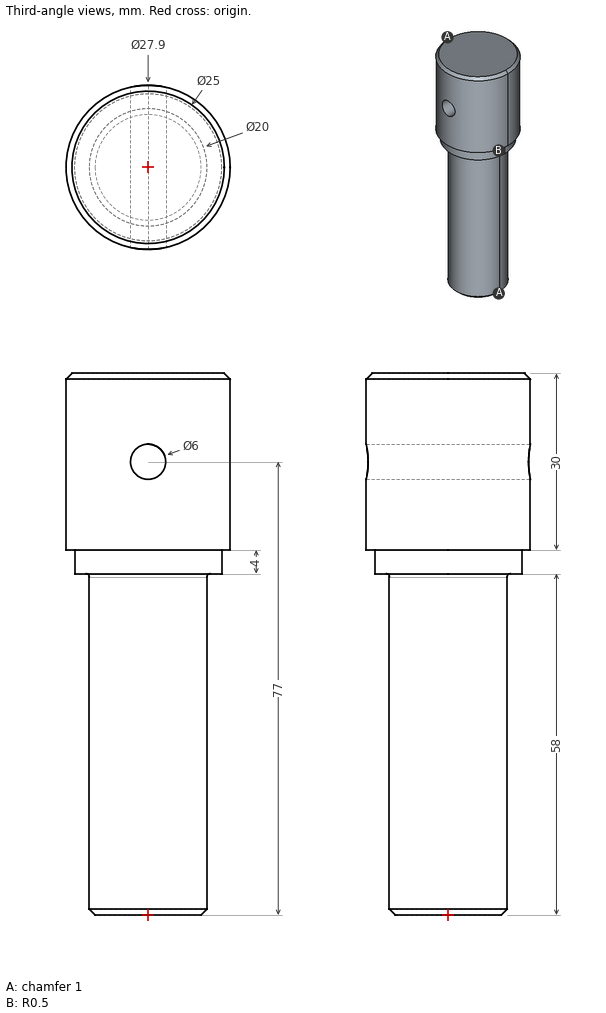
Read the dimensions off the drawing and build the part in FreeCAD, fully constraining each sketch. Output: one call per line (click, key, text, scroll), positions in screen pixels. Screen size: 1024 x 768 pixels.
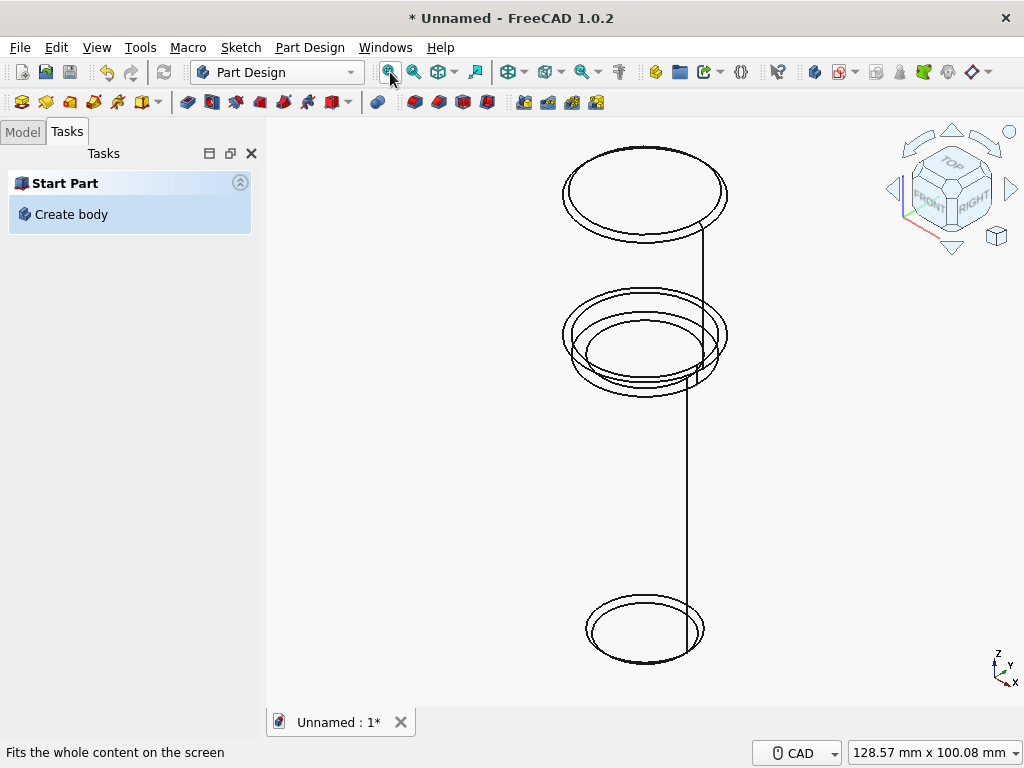
click(603, 329)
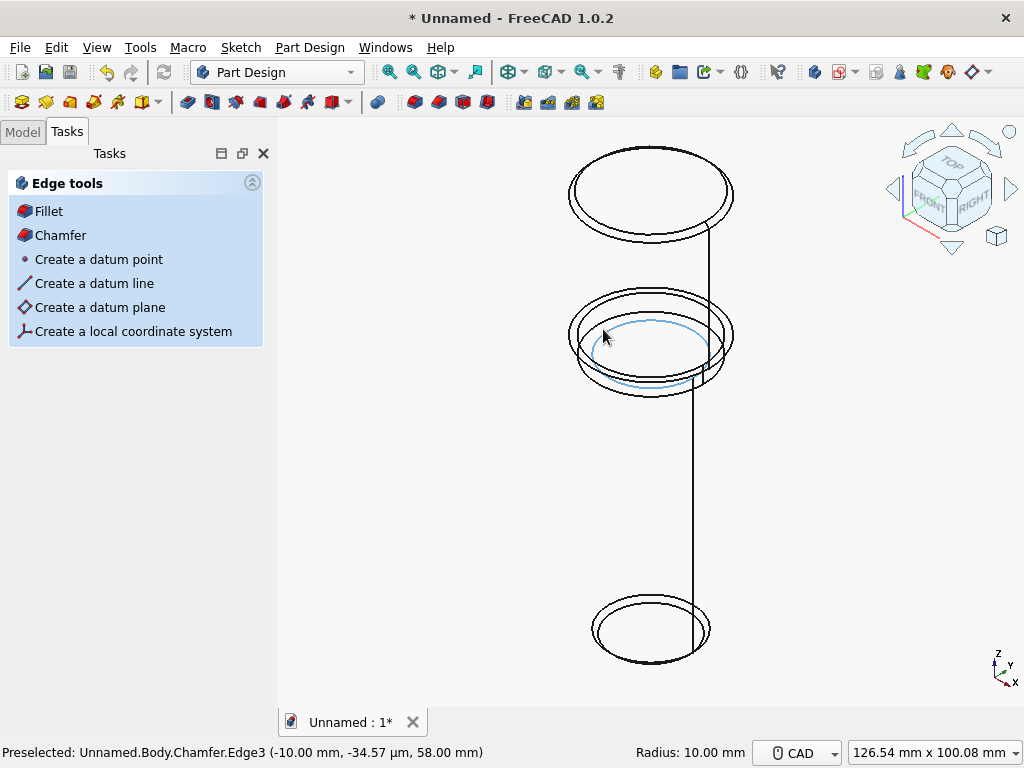
key(v)
key(1)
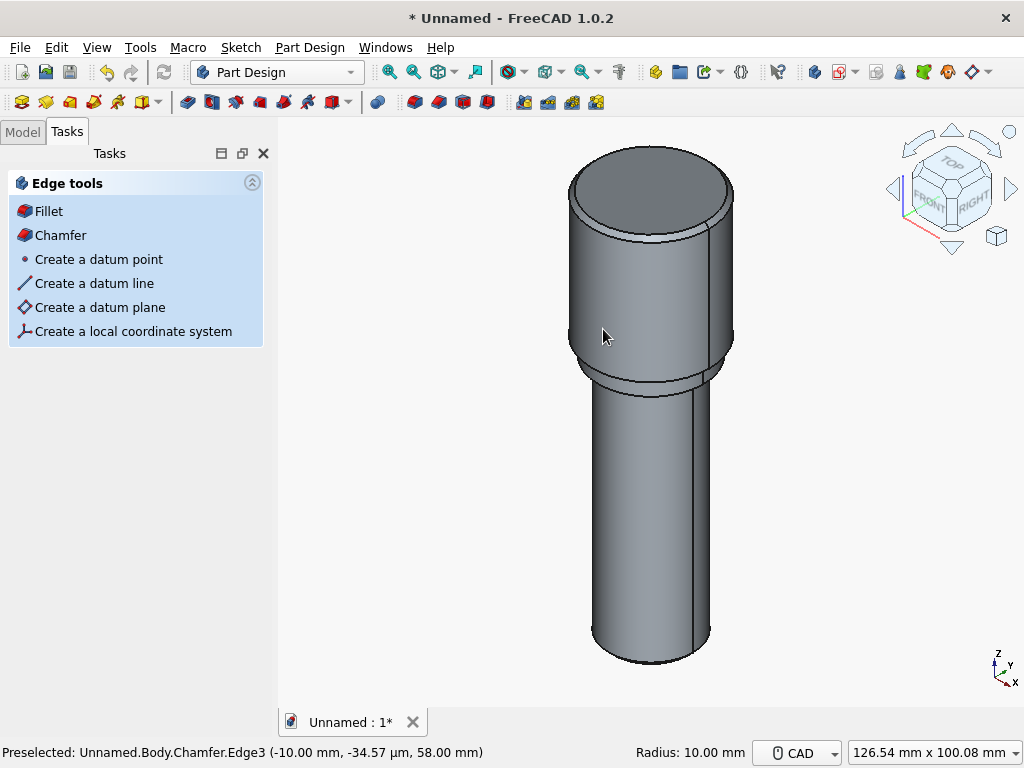
click(416, 102)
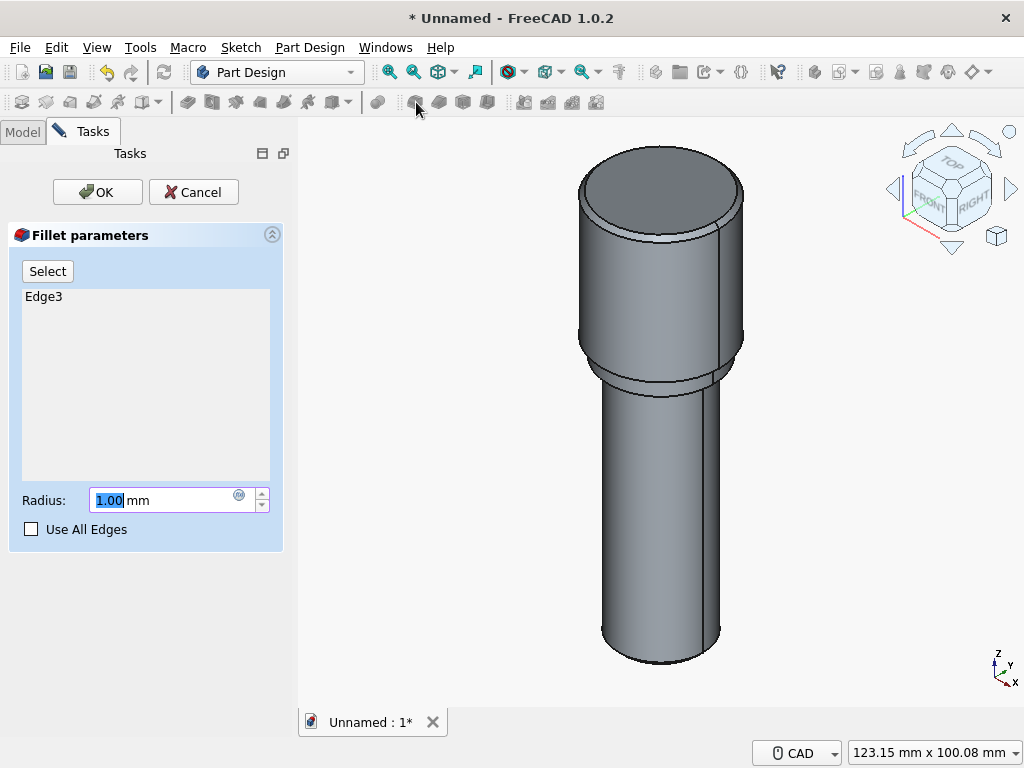
text(0.5)
key(Tab)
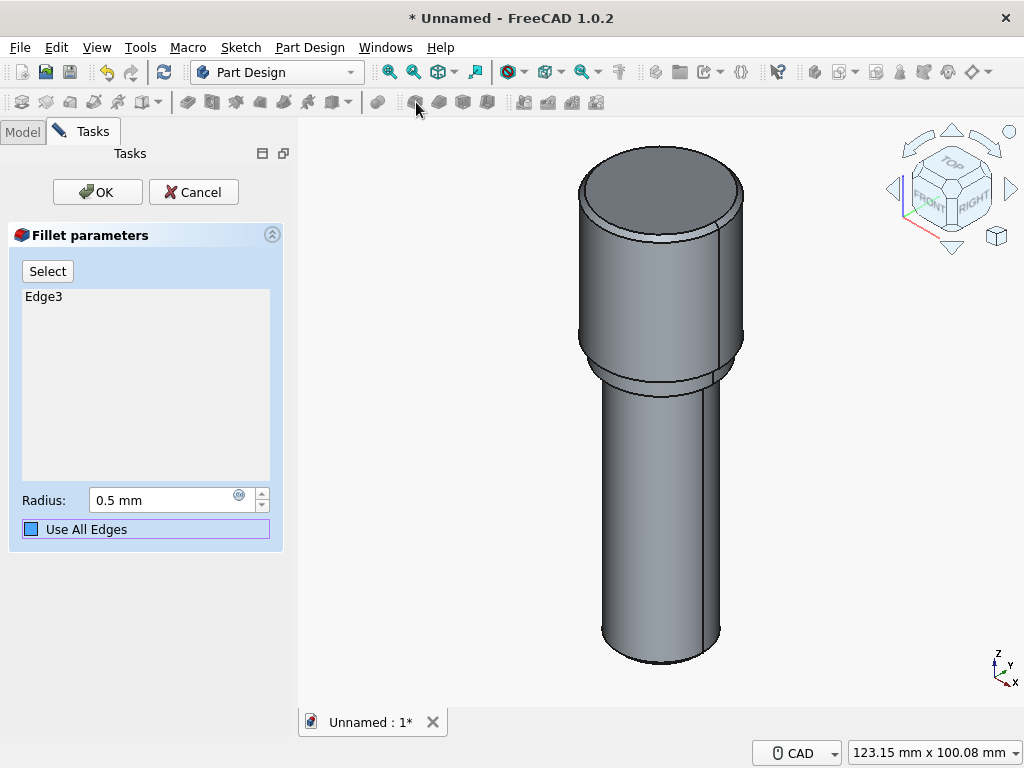
click(98, 192)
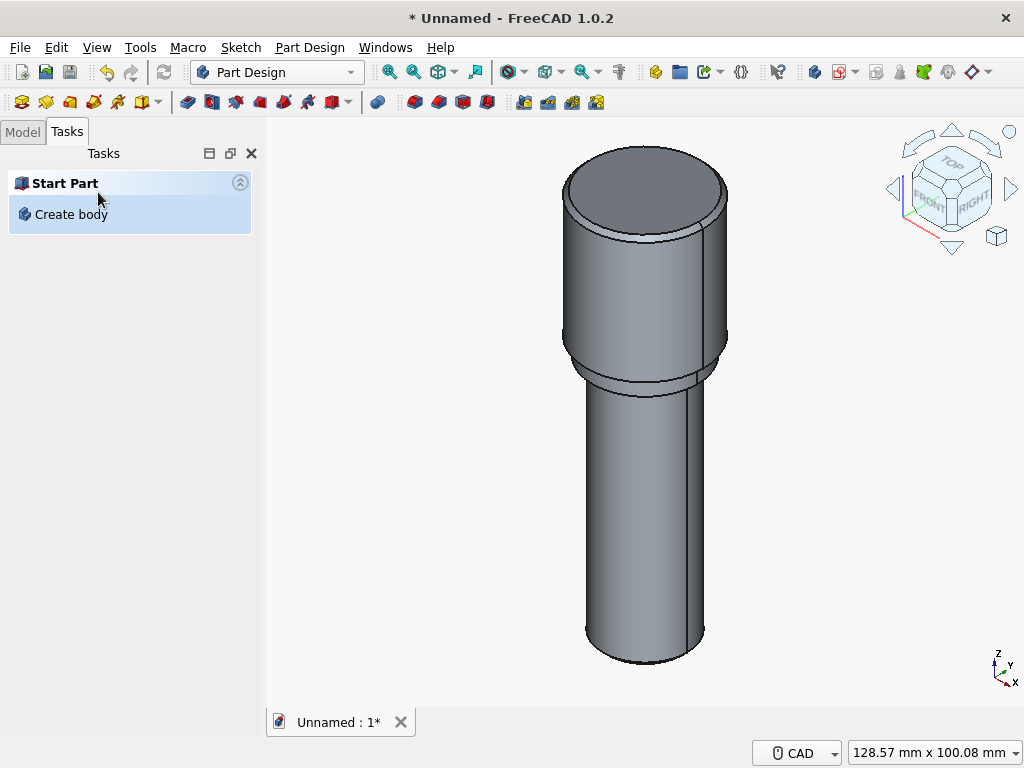
click(840, 72)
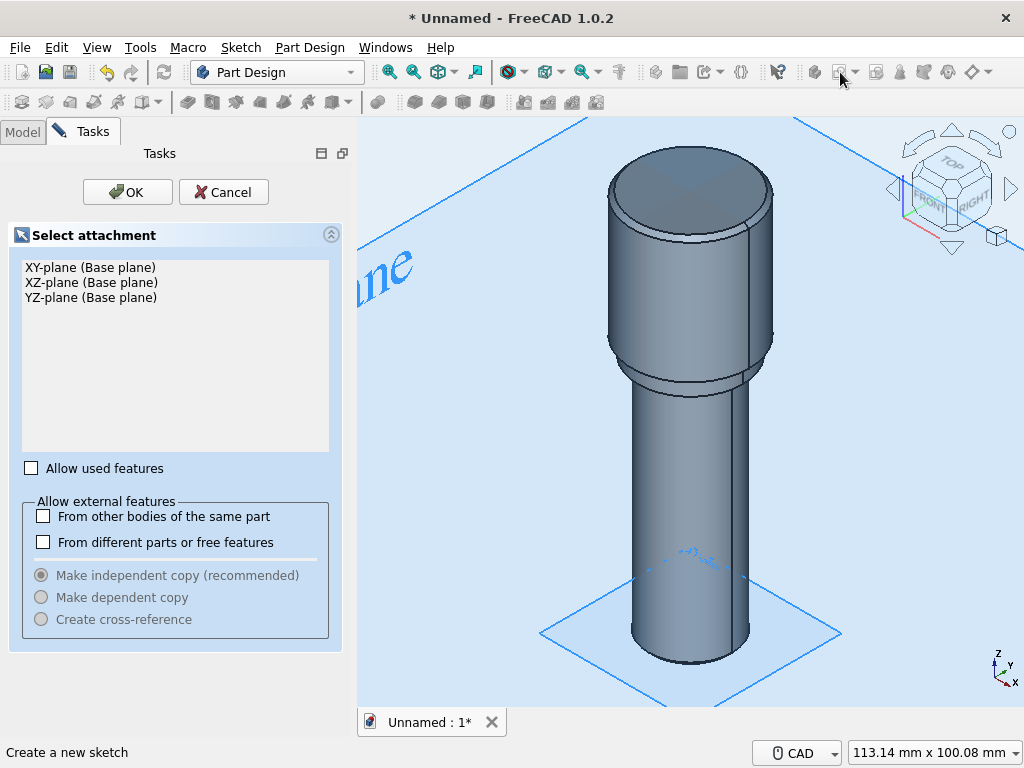
click(82, 282)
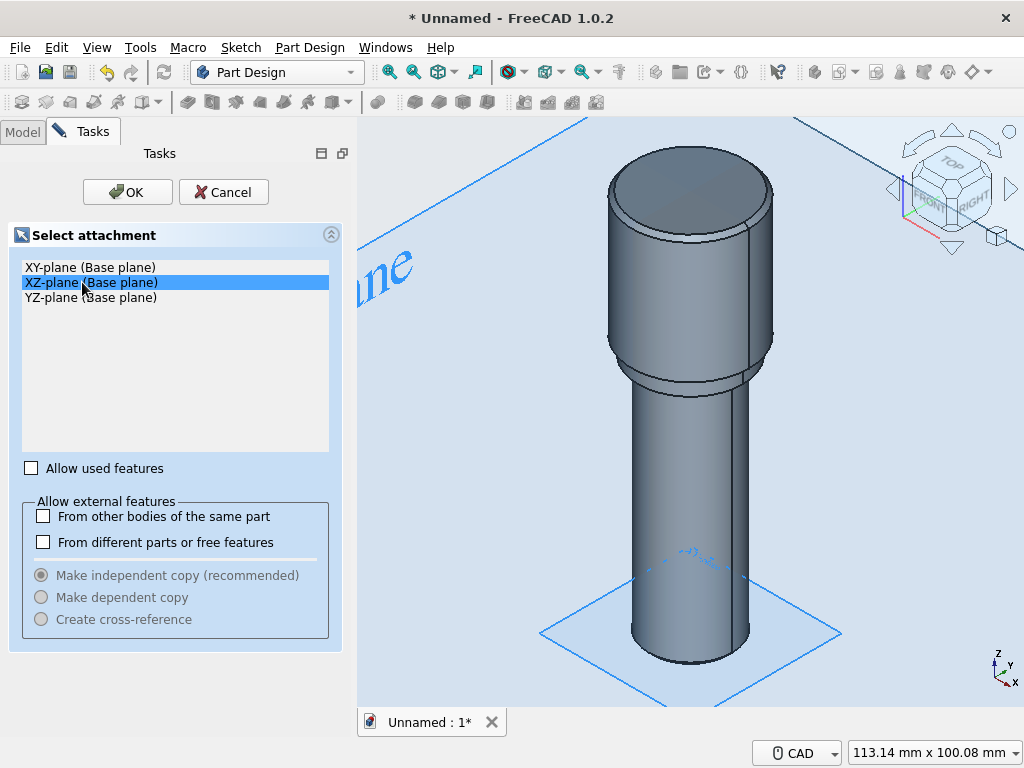
click(128, 192)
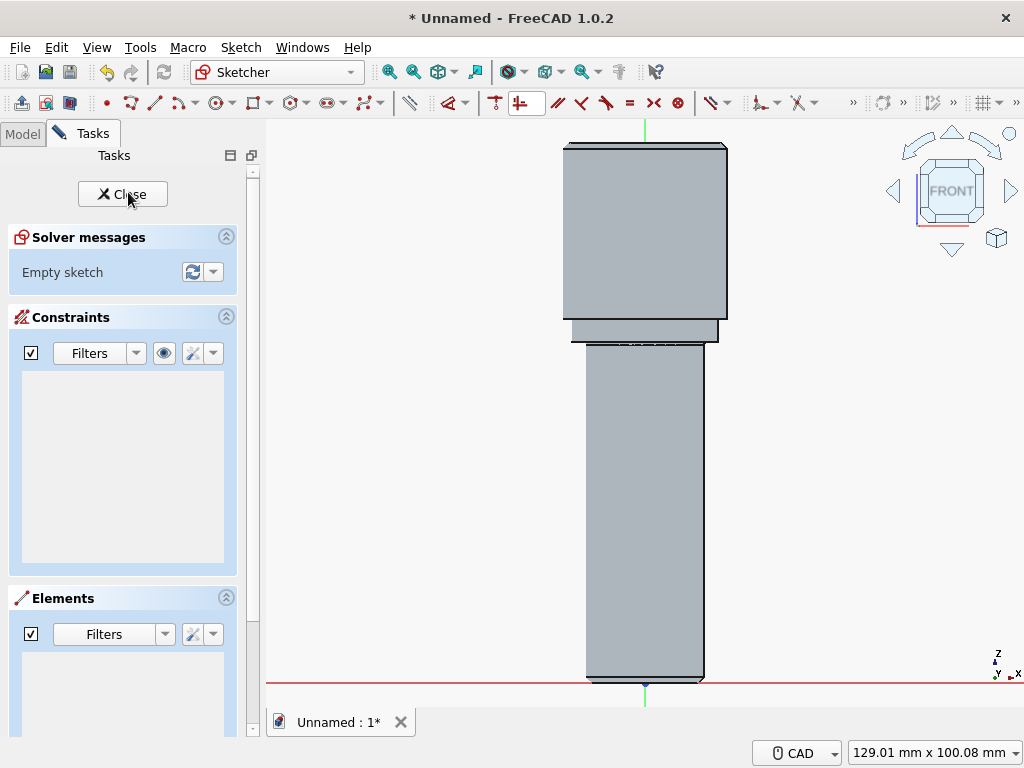
click(70, 104)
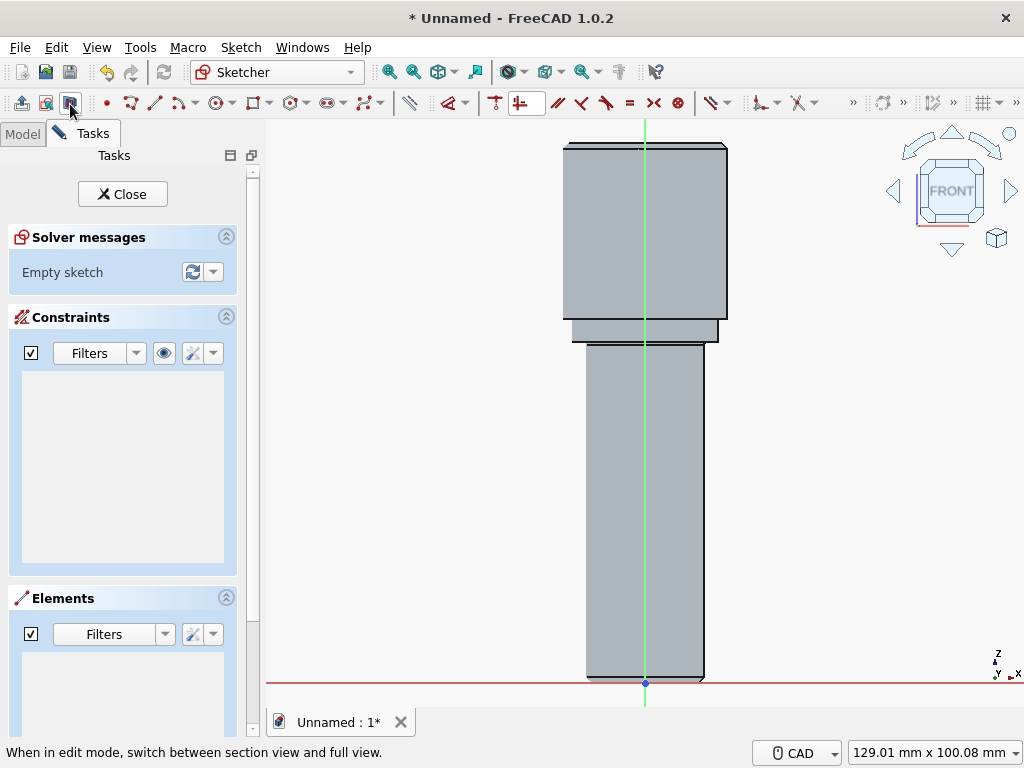
scroll(652, 213, up, 12)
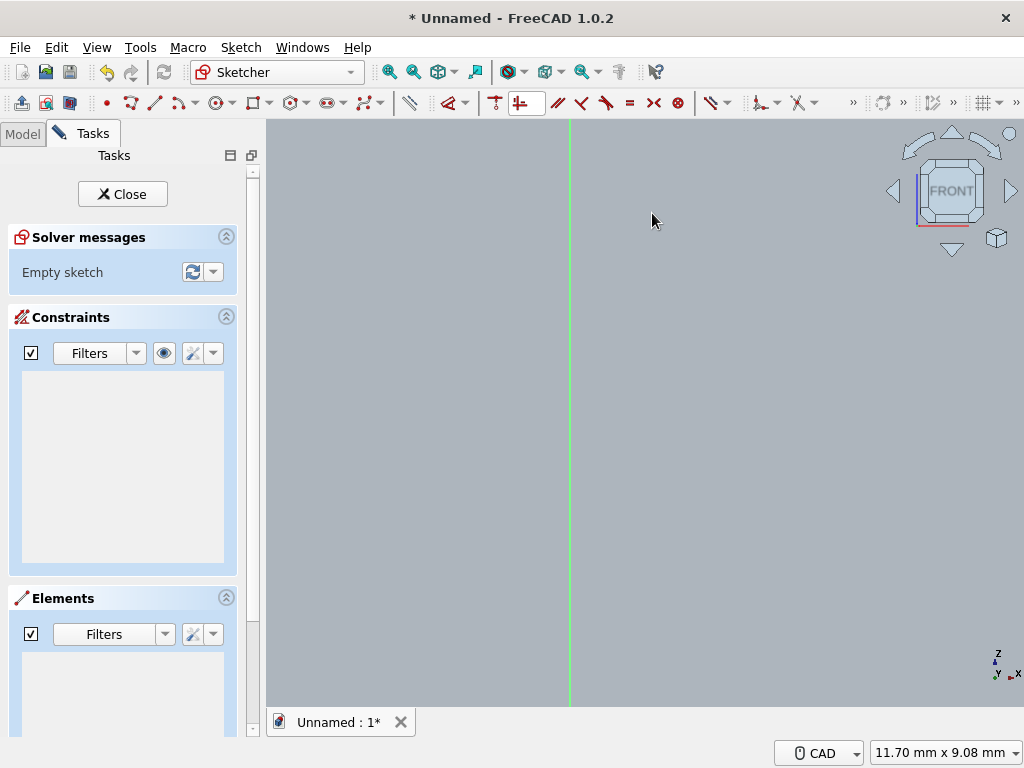
click(216, 104)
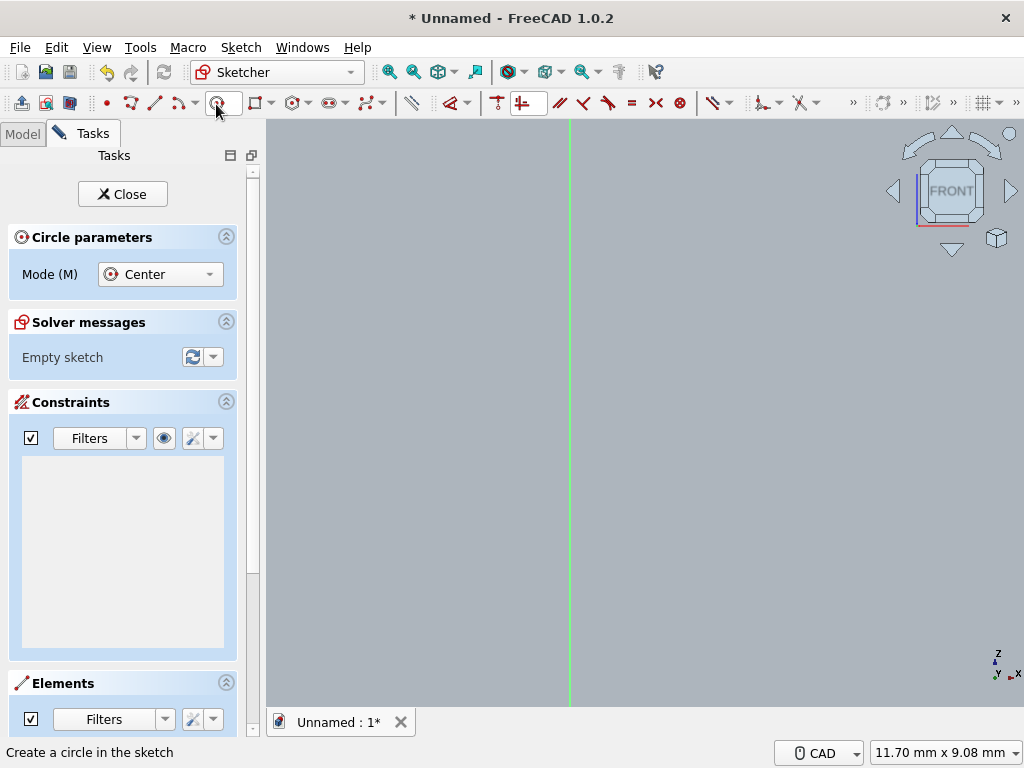
click(570, 408)
click(707, 271)
key(Escape)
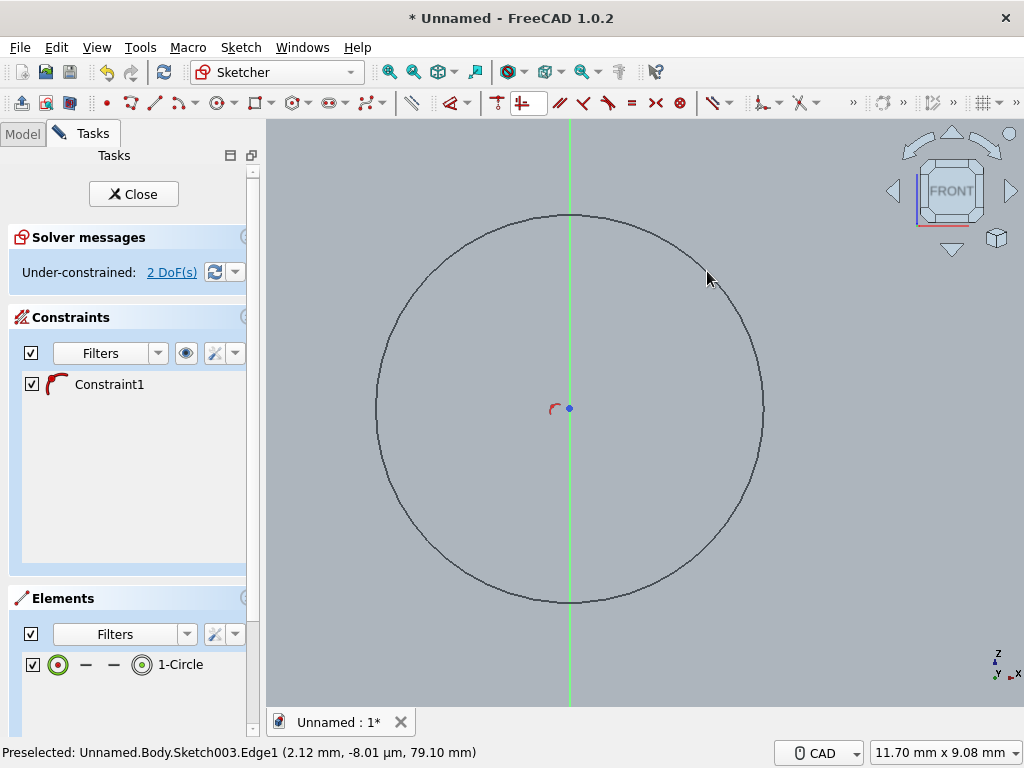
click(450, 104)